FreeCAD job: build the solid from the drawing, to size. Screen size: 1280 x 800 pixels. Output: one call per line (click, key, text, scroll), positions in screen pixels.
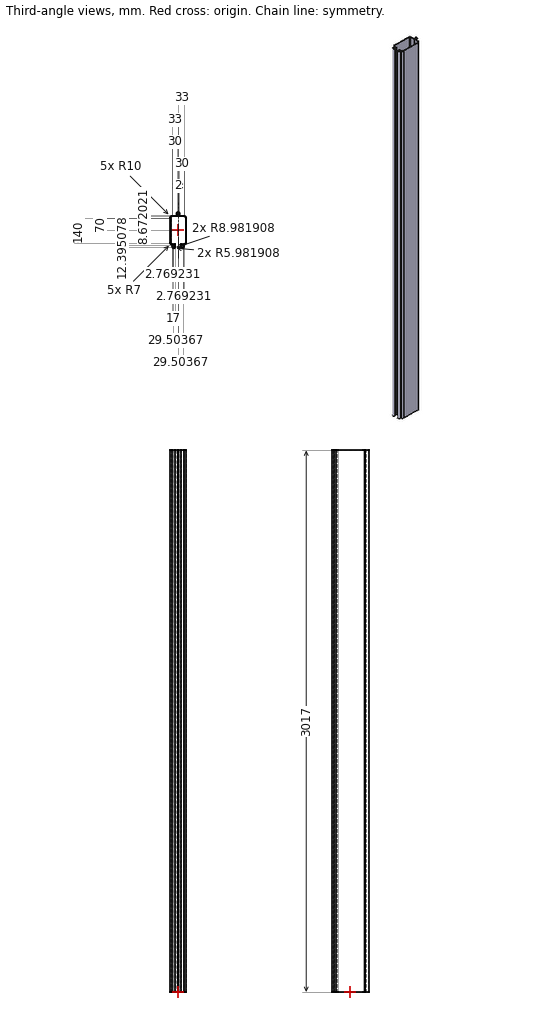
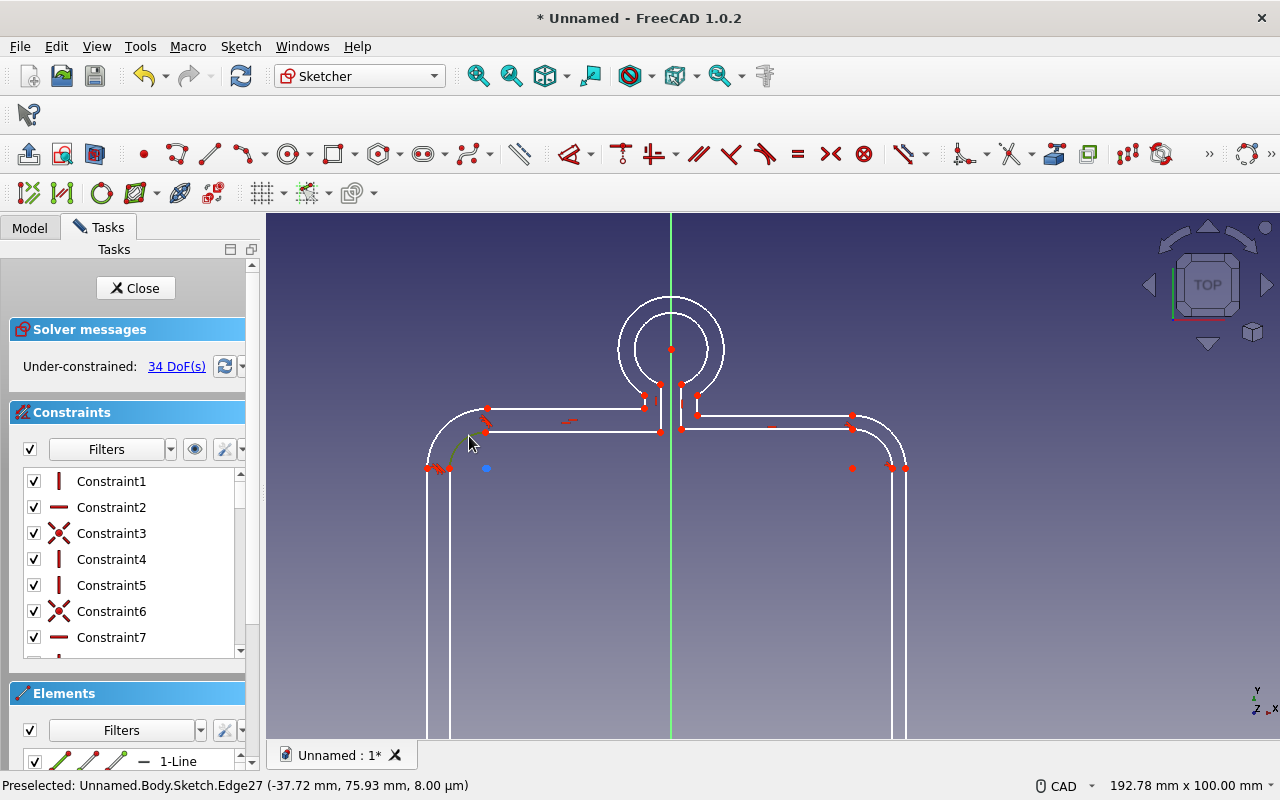
click(460, 416)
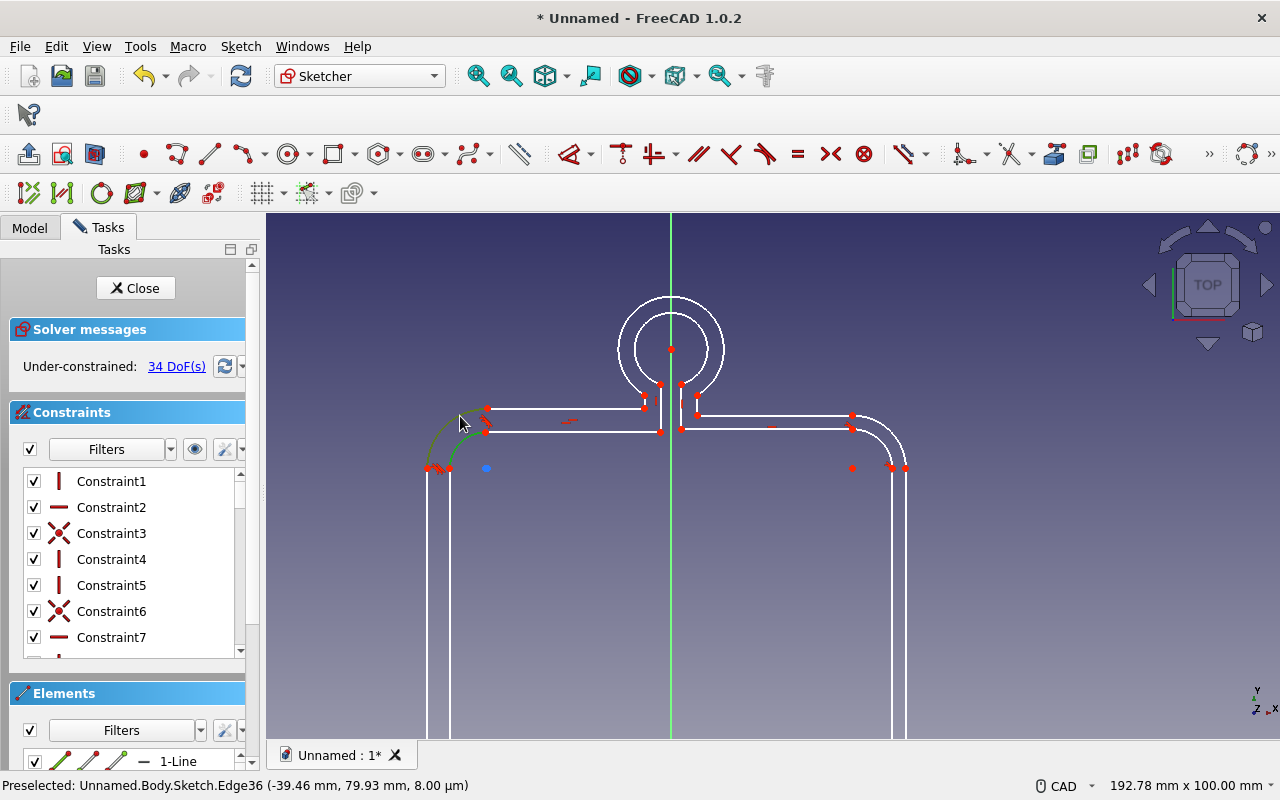
click(621, 154)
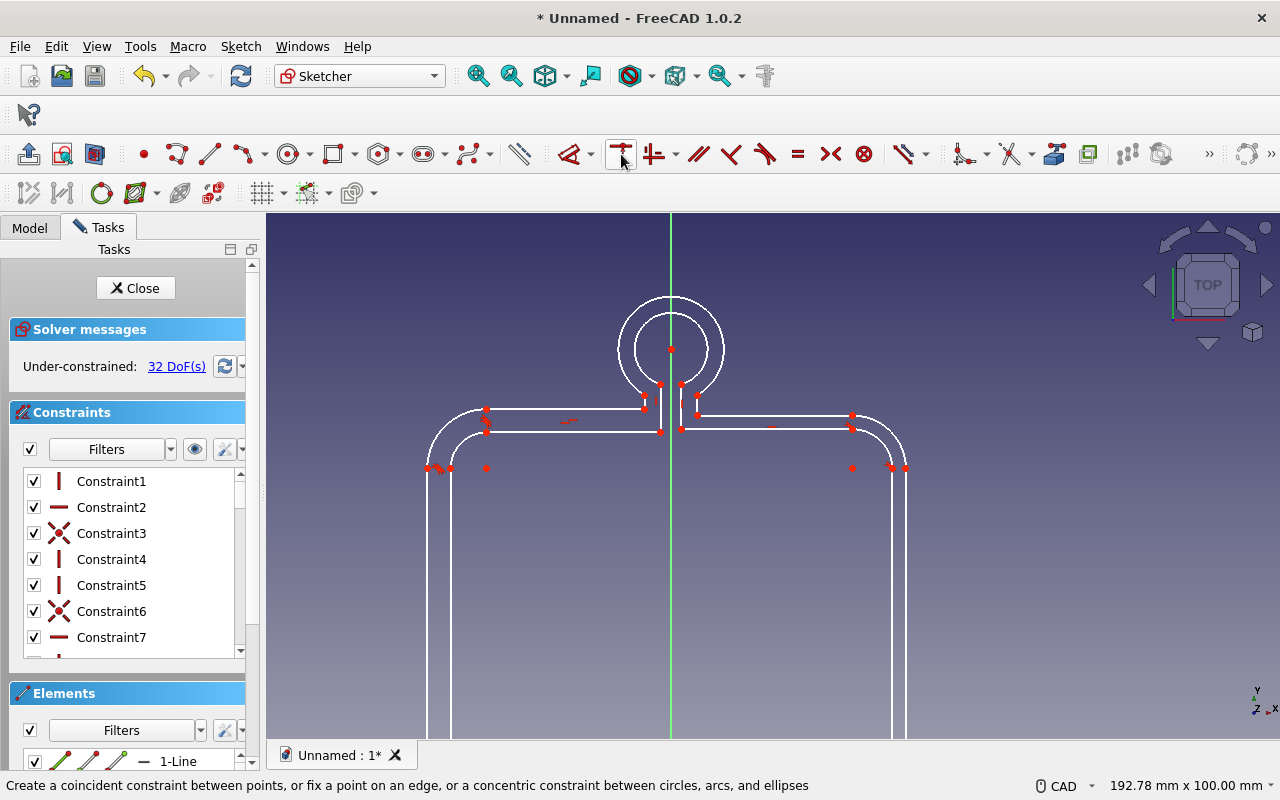
scroll(719, 323, down, 6)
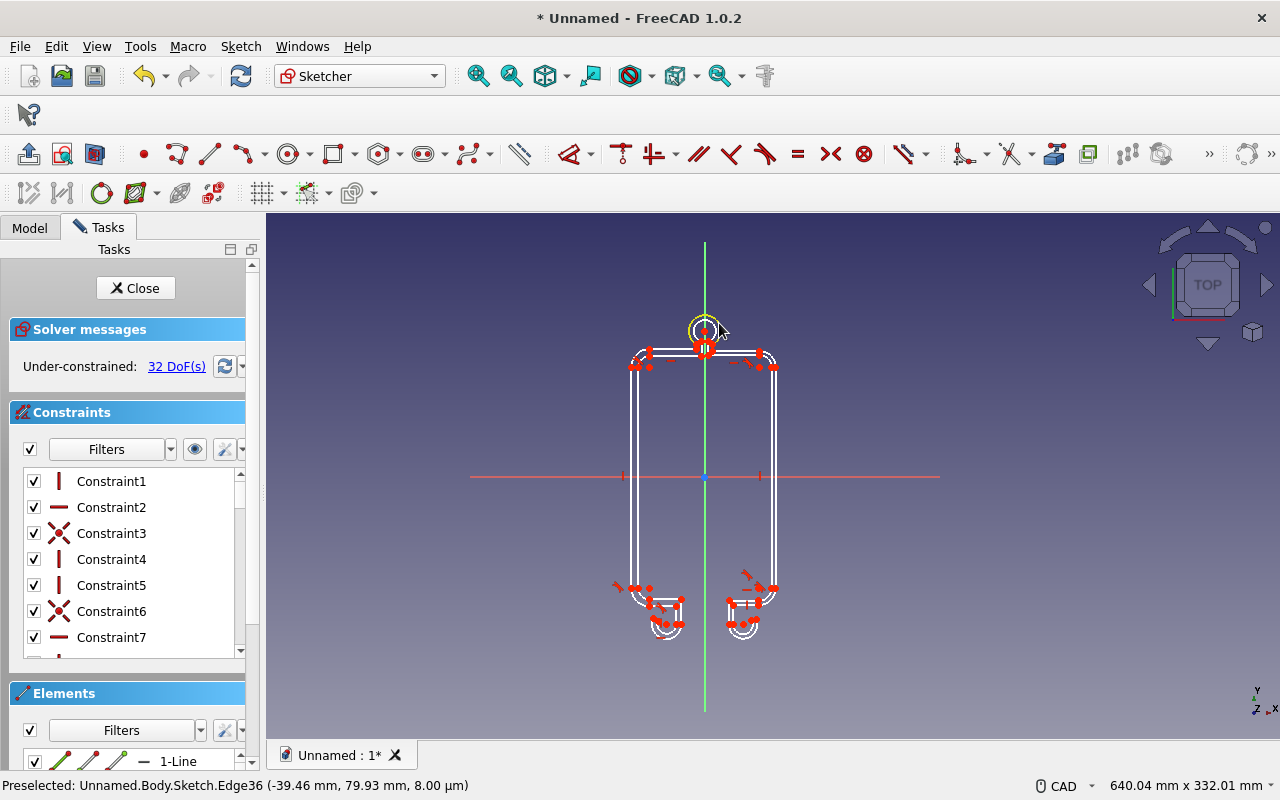
scroll(640, 593, up, 5)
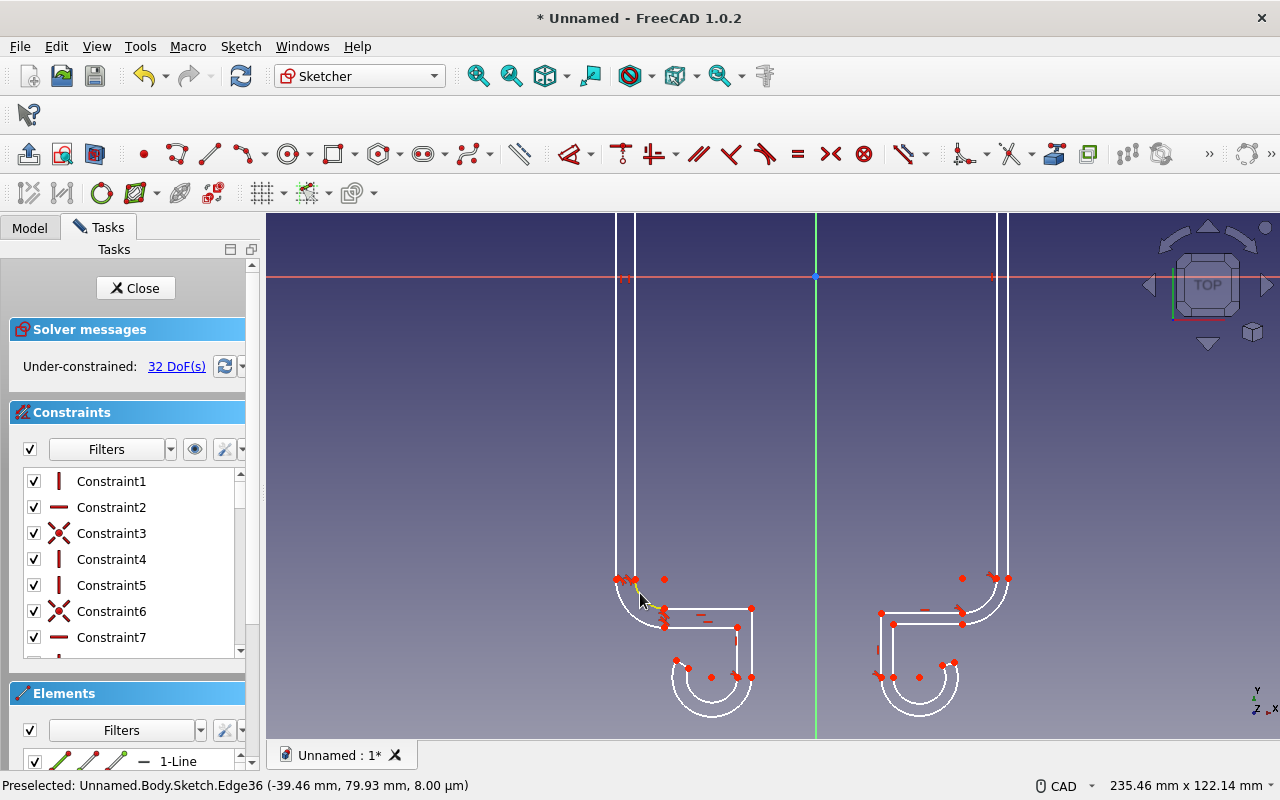
click(638, 592)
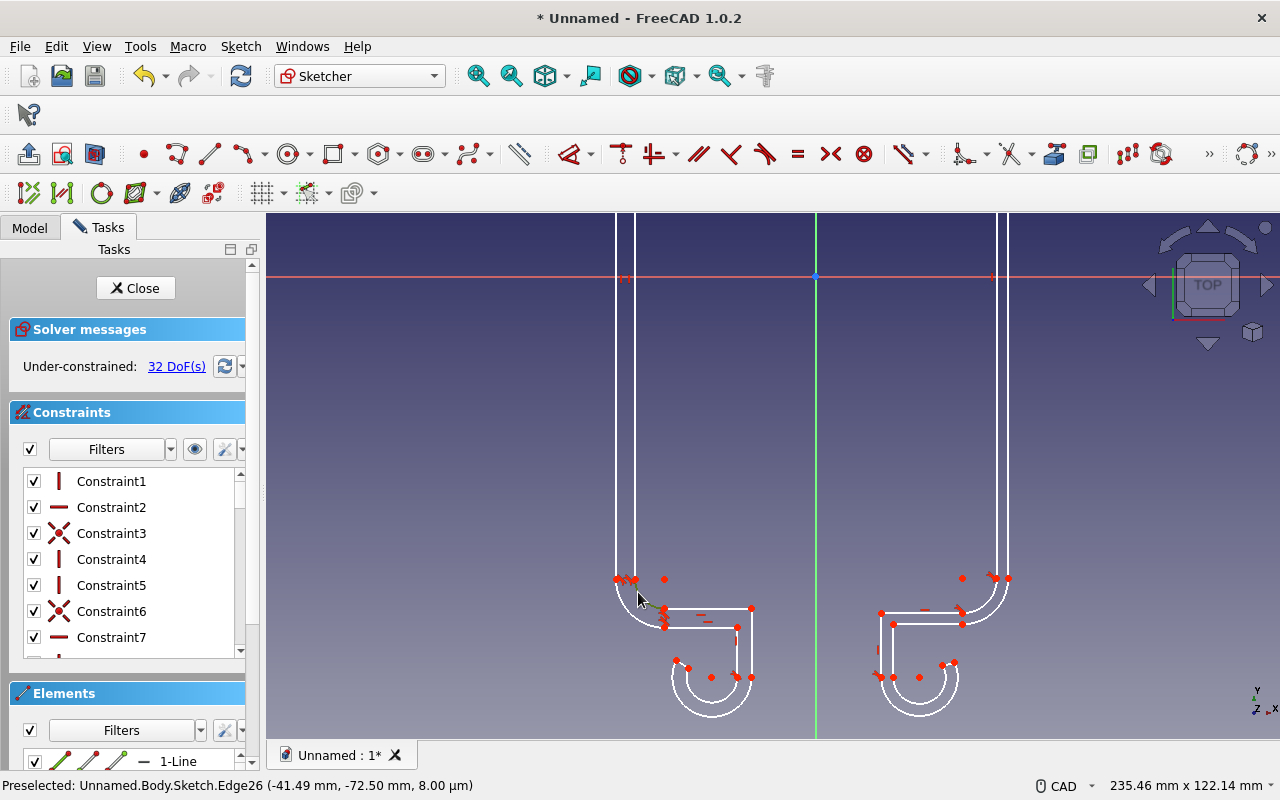
scroll(640, 593, down, 5)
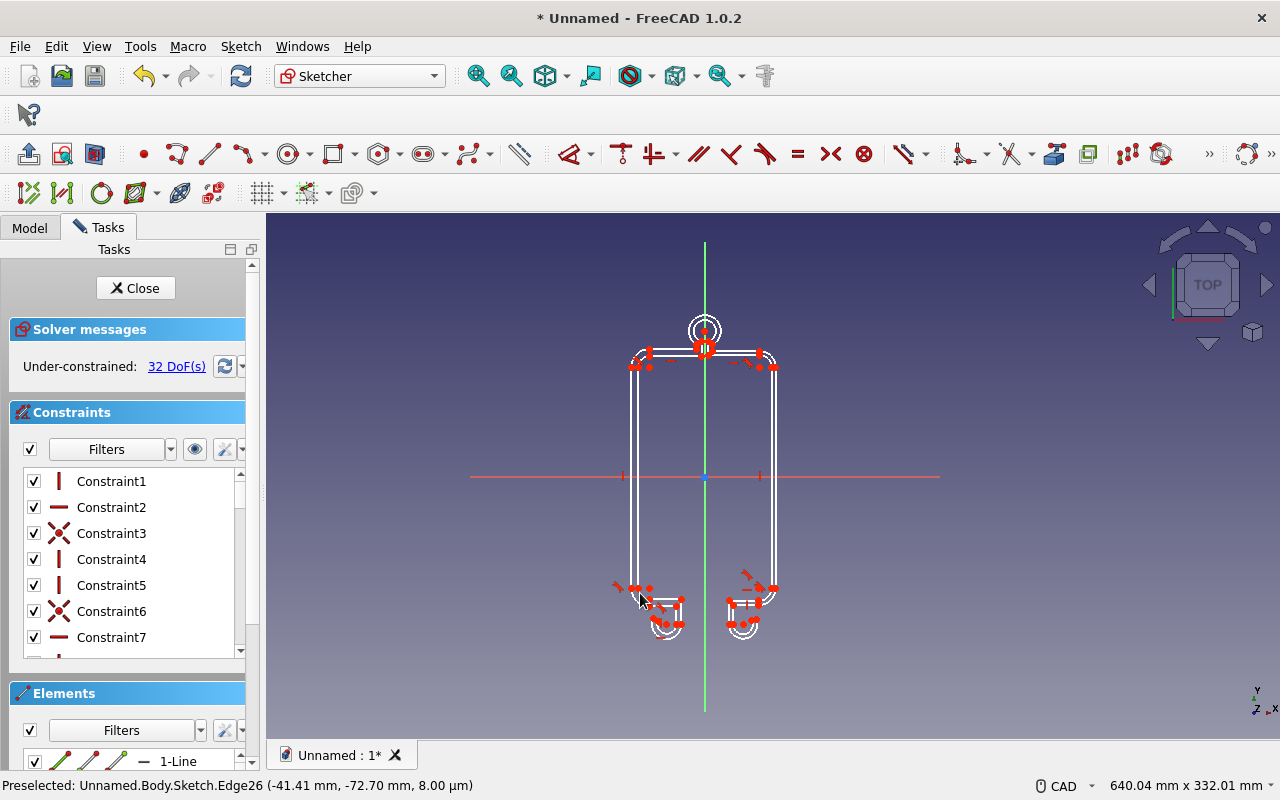
scroll(644, 357, up, 5)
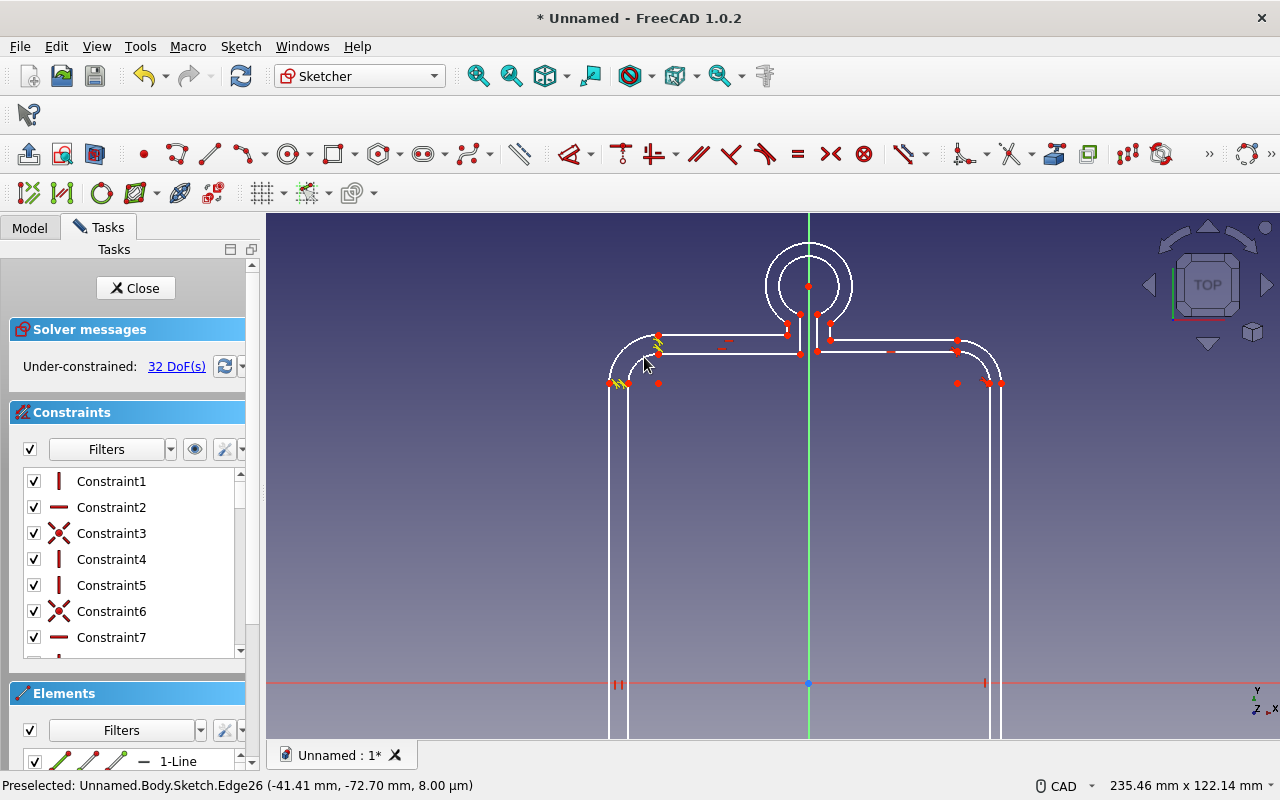
click(645, 357)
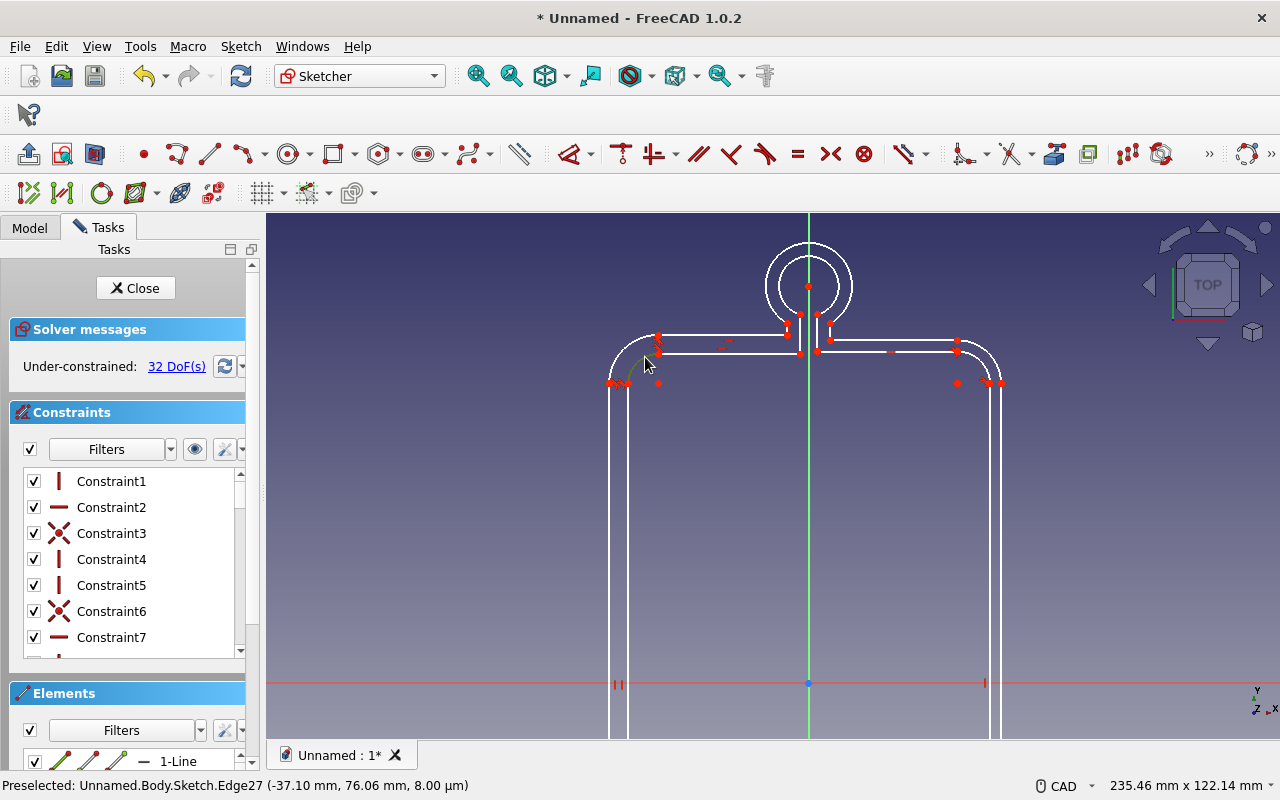
click(836, 274)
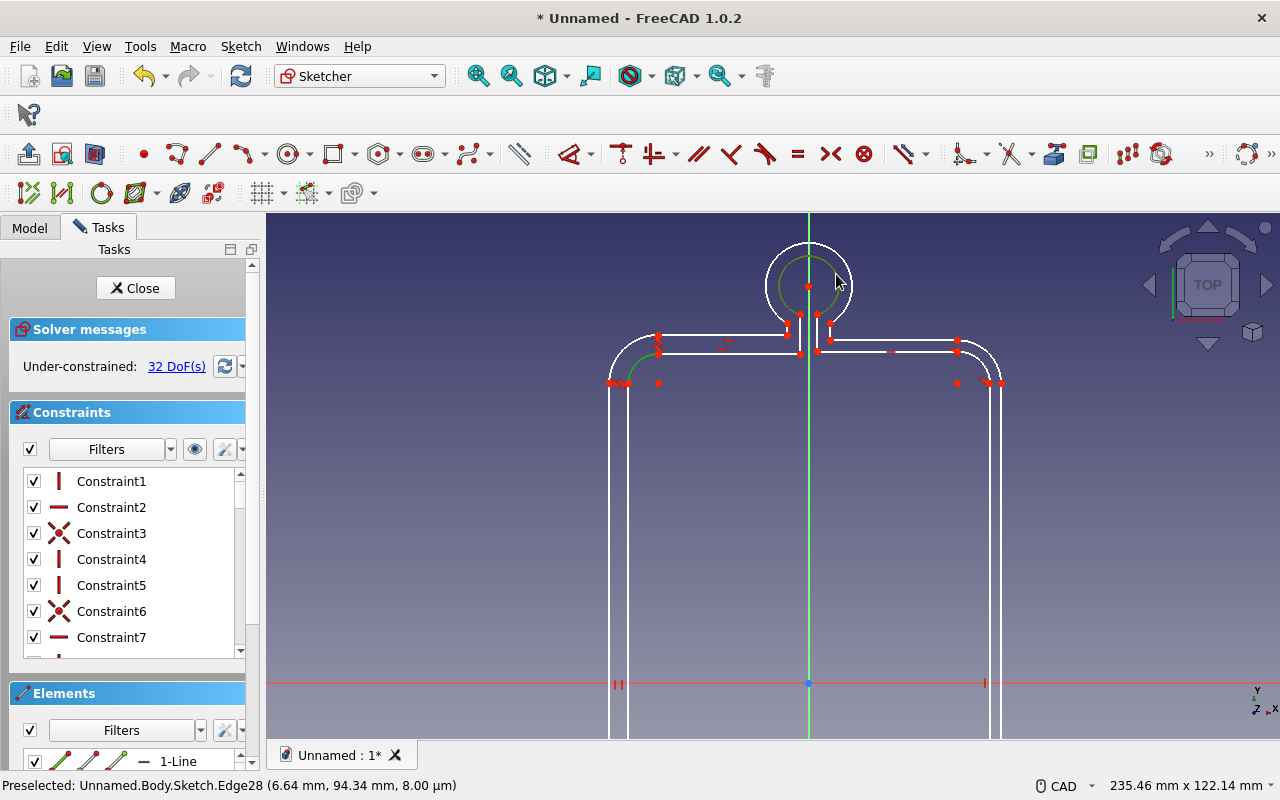
scroll(986, 369, up, 2)